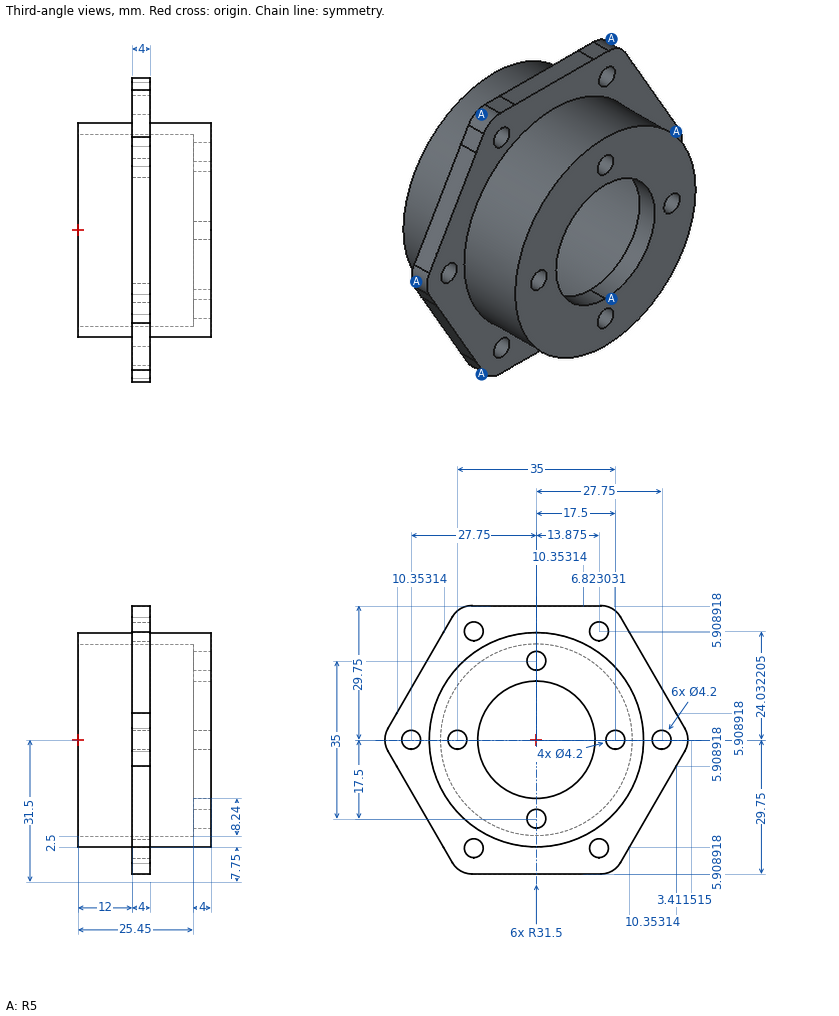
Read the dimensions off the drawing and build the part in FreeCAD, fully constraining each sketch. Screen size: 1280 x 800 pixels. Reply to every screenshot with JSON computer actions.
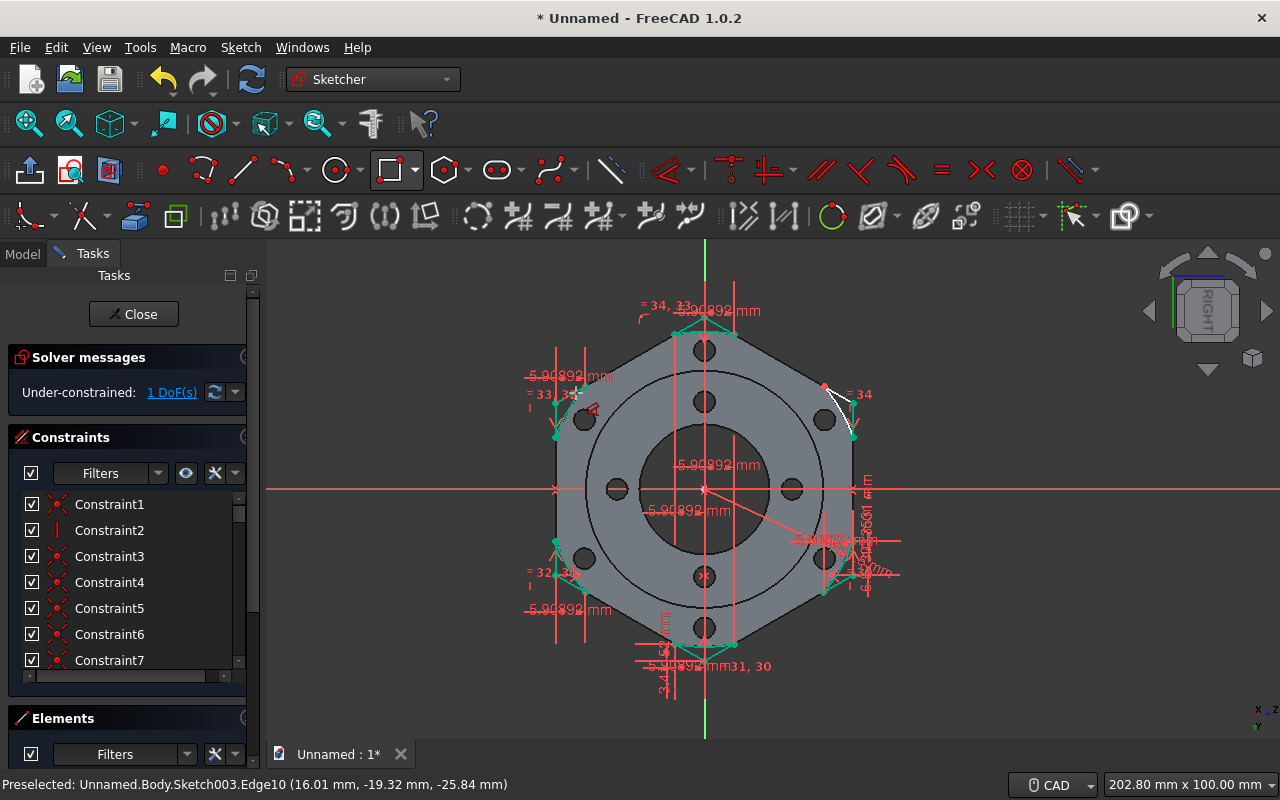
{"action": "scroll", "coordinate": [844, 398], "scroll_direction": "up", "scroll_amount": 2}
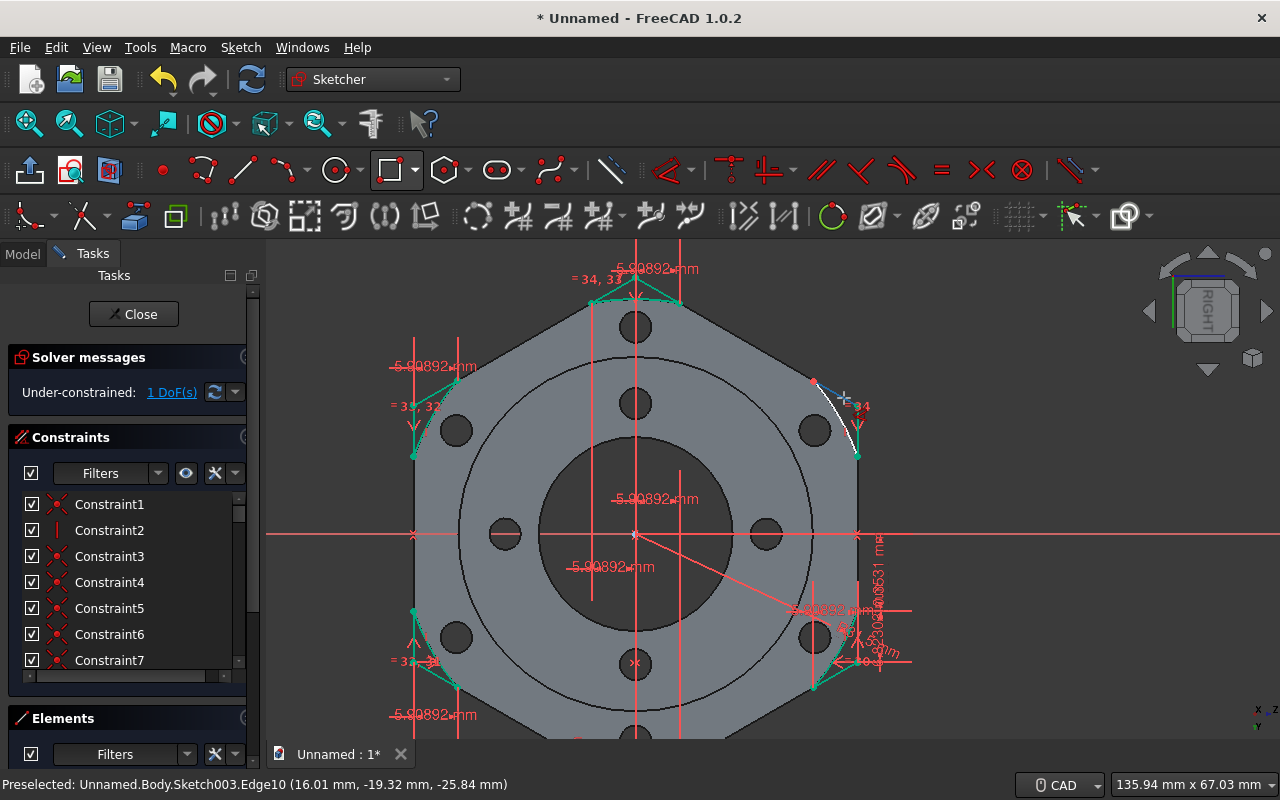
{"action": "left_click", "coordinate": [844, 398]}
{"action": "left_click", "coordinate": [836, 347]}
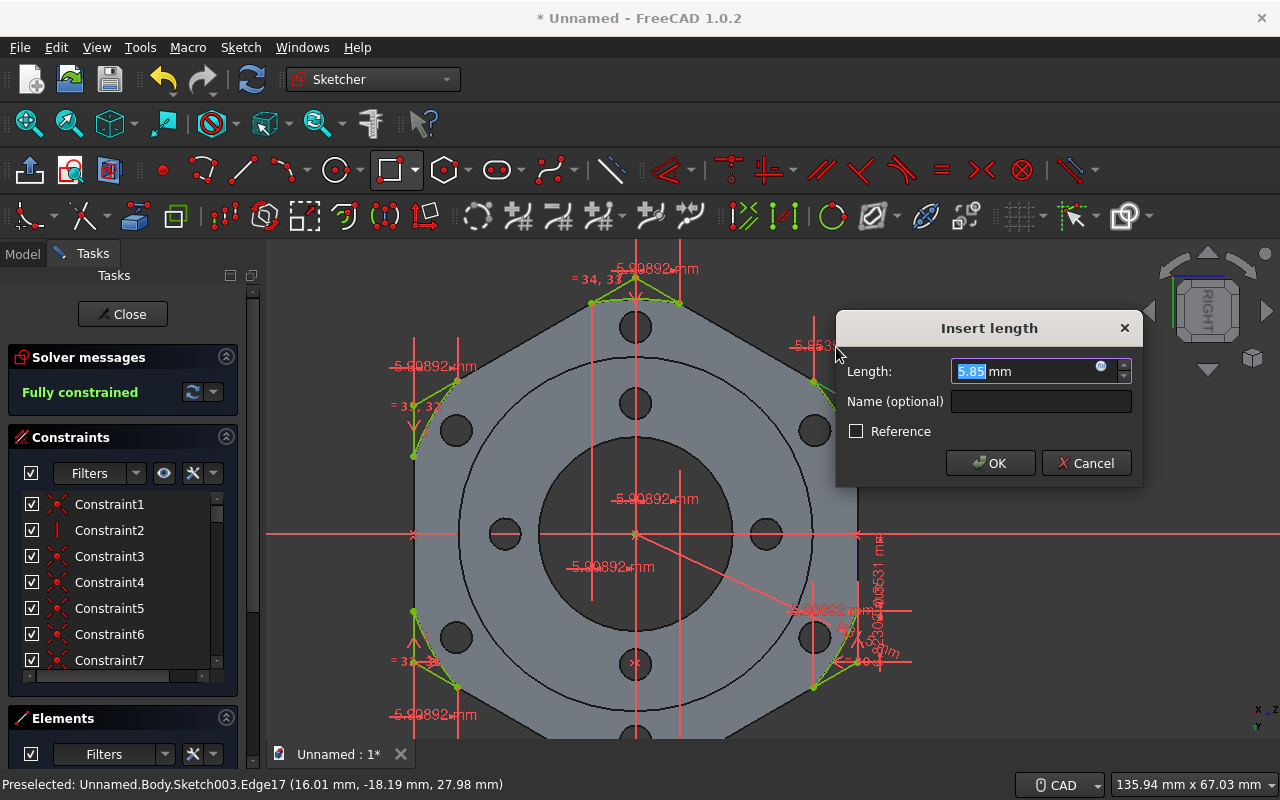
{"action": "type", "text": "5.908918"}
{"action": "key", "text": "Return"}
{"action": "key", "text": "Escape"}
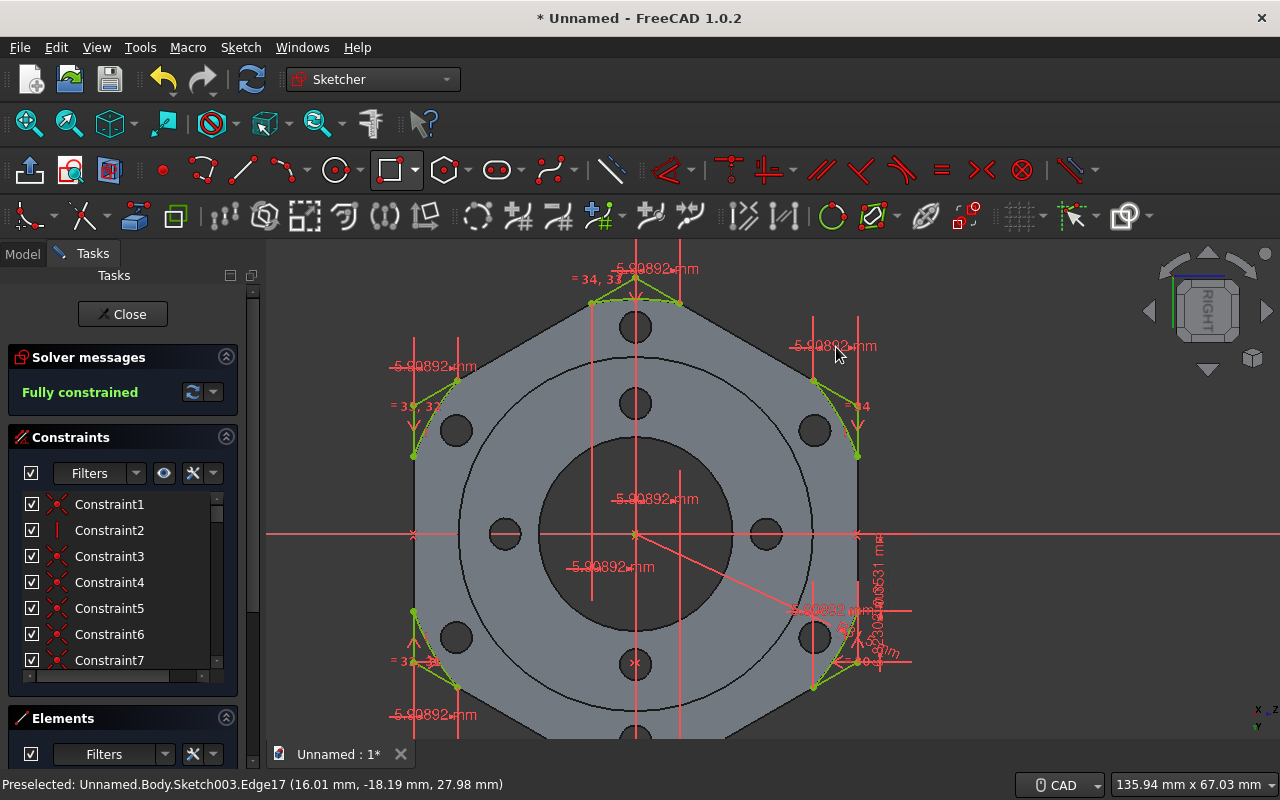
{"action": "left_click", "coordinate": [123, 314]}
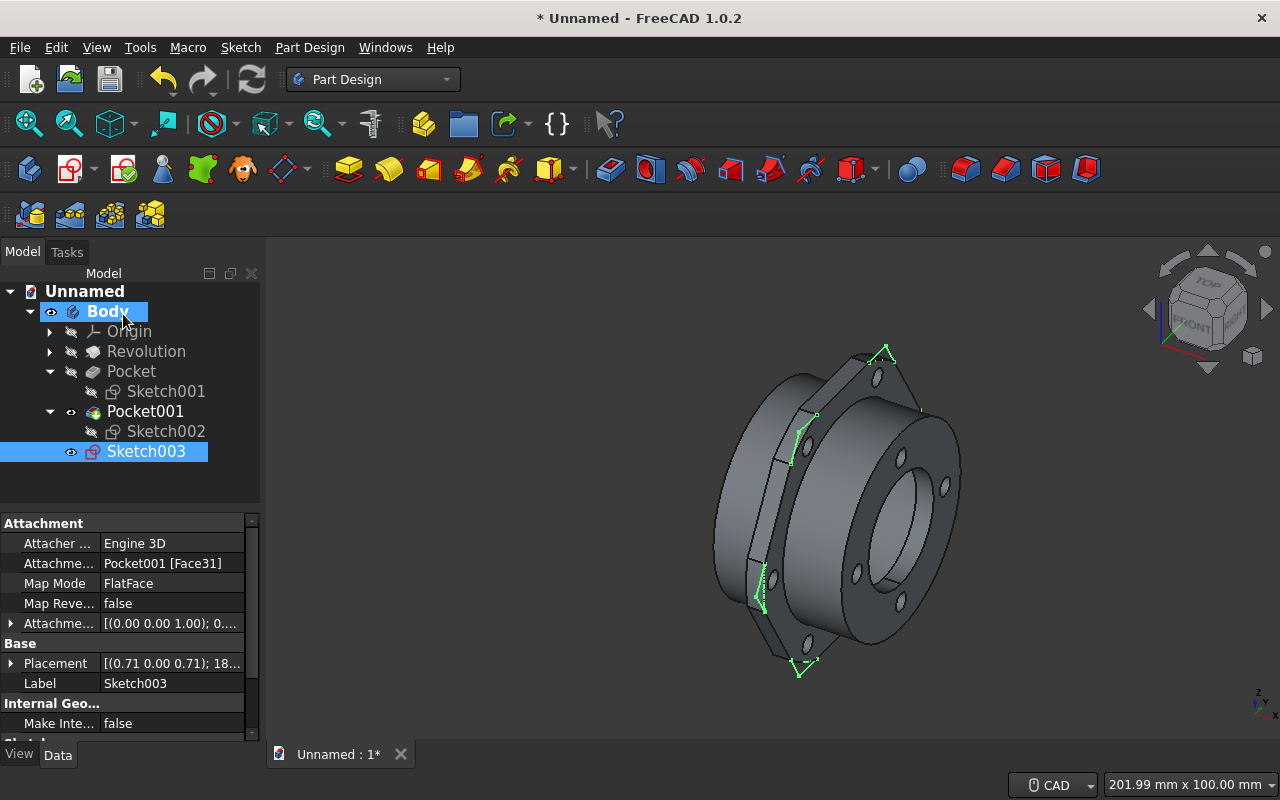
{"action": "left_click", "coordinate": [350, 170]}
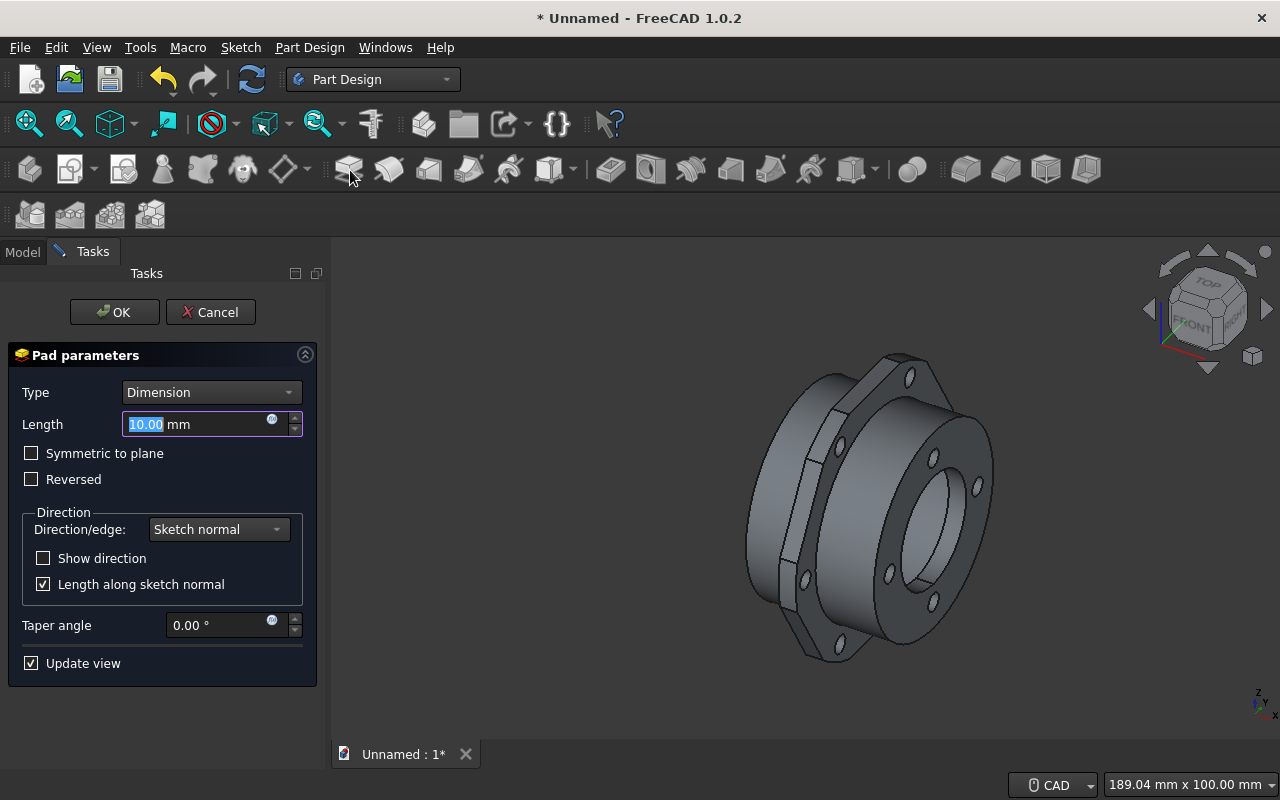
{"action": "type", "text": "4"}
{"action": "key", "text": "Tab"}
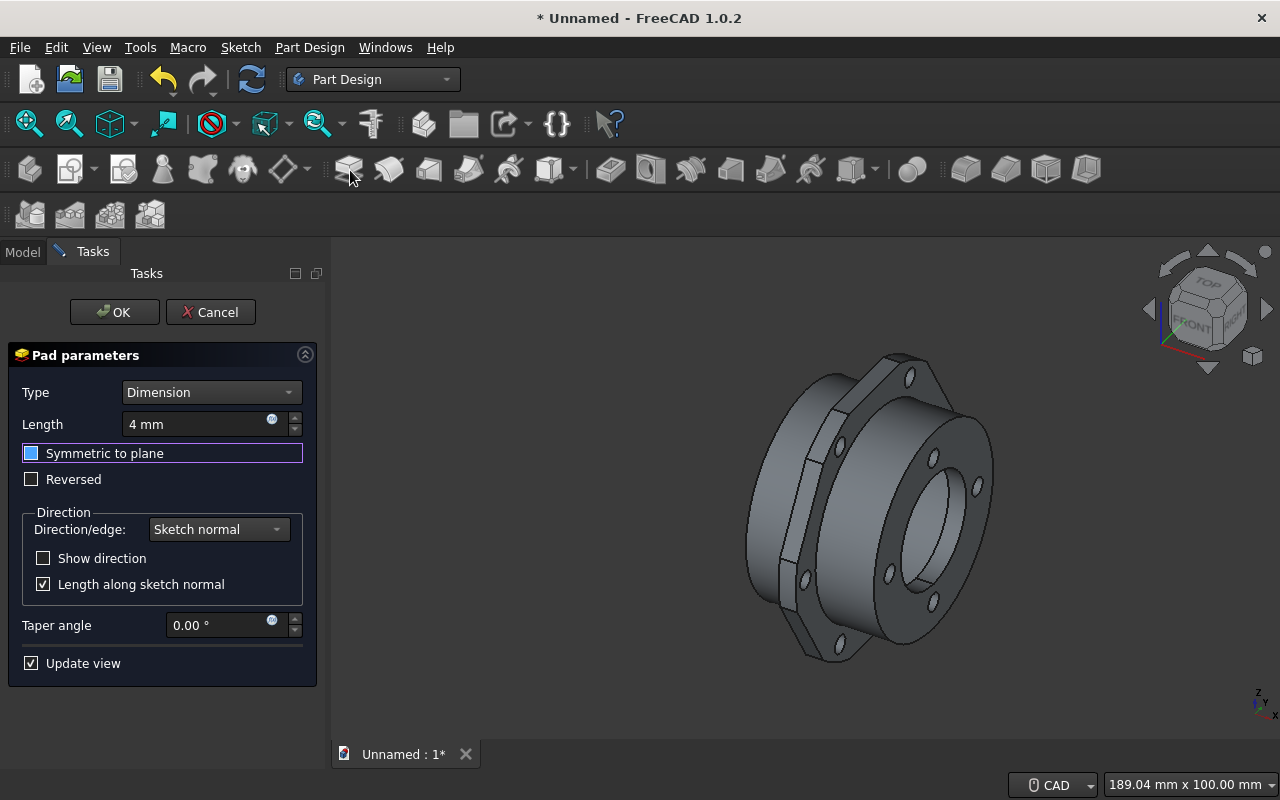
{"action": "left_click", "coordinate": [30, 479]}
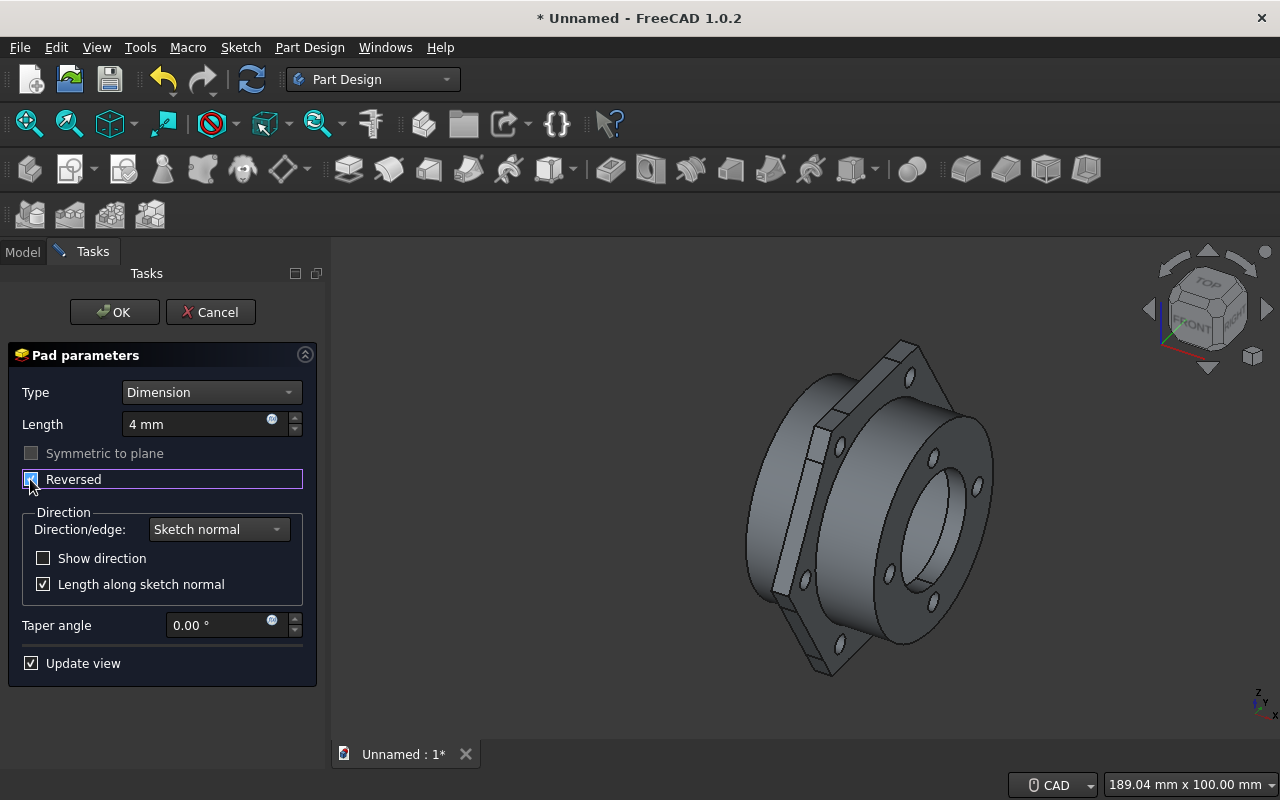
{"action": "left_click", "coordinate": [115, 312]}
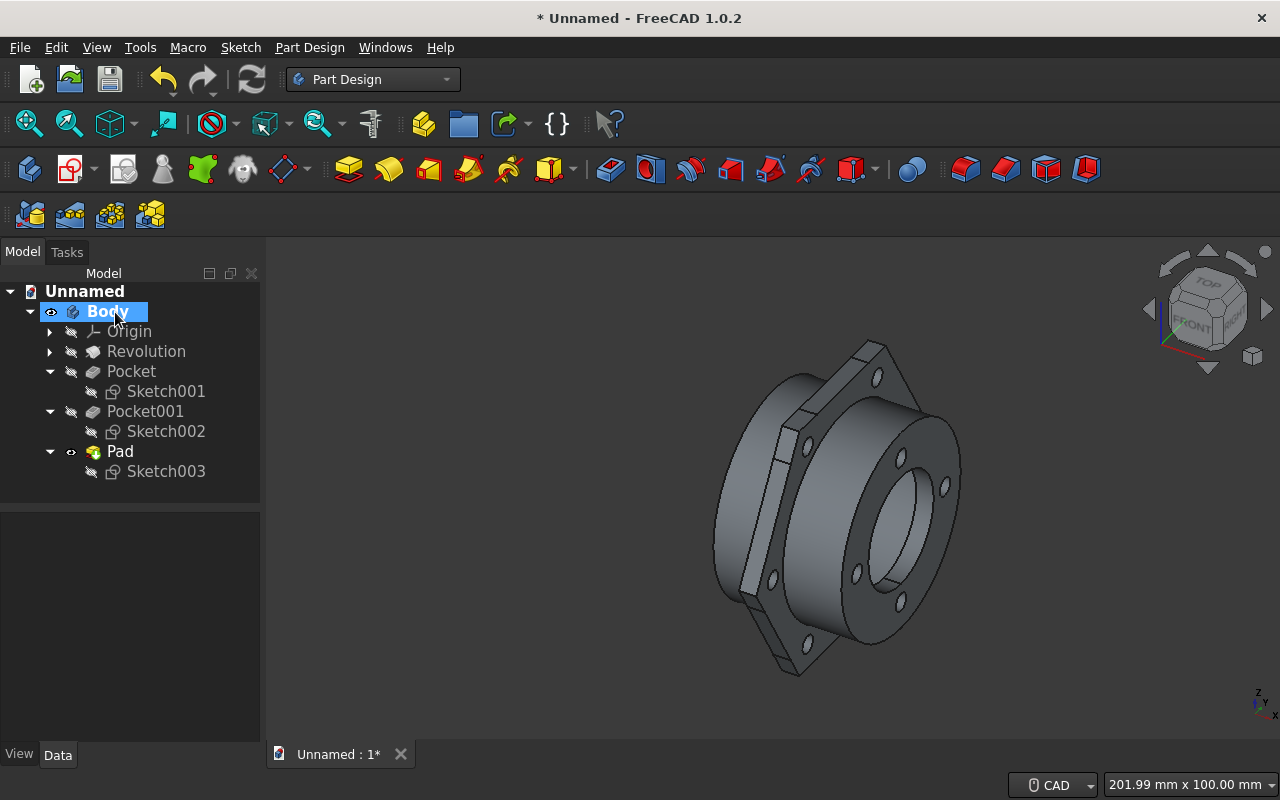
{"action": "left_click", "coordinate": [791, 428]}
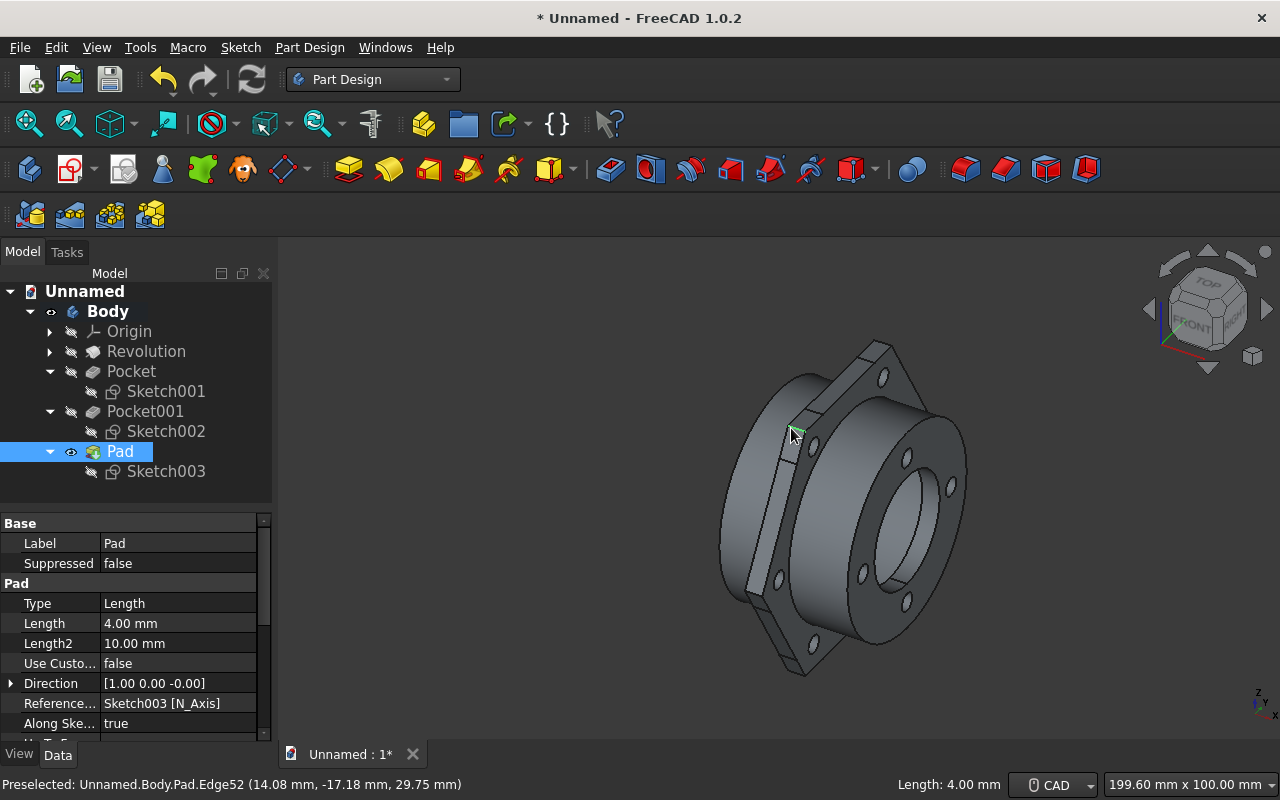
{"action": "scroll", "coordinate": [754, 593], "scroll_direction": "up", "scroll_amount": 4}